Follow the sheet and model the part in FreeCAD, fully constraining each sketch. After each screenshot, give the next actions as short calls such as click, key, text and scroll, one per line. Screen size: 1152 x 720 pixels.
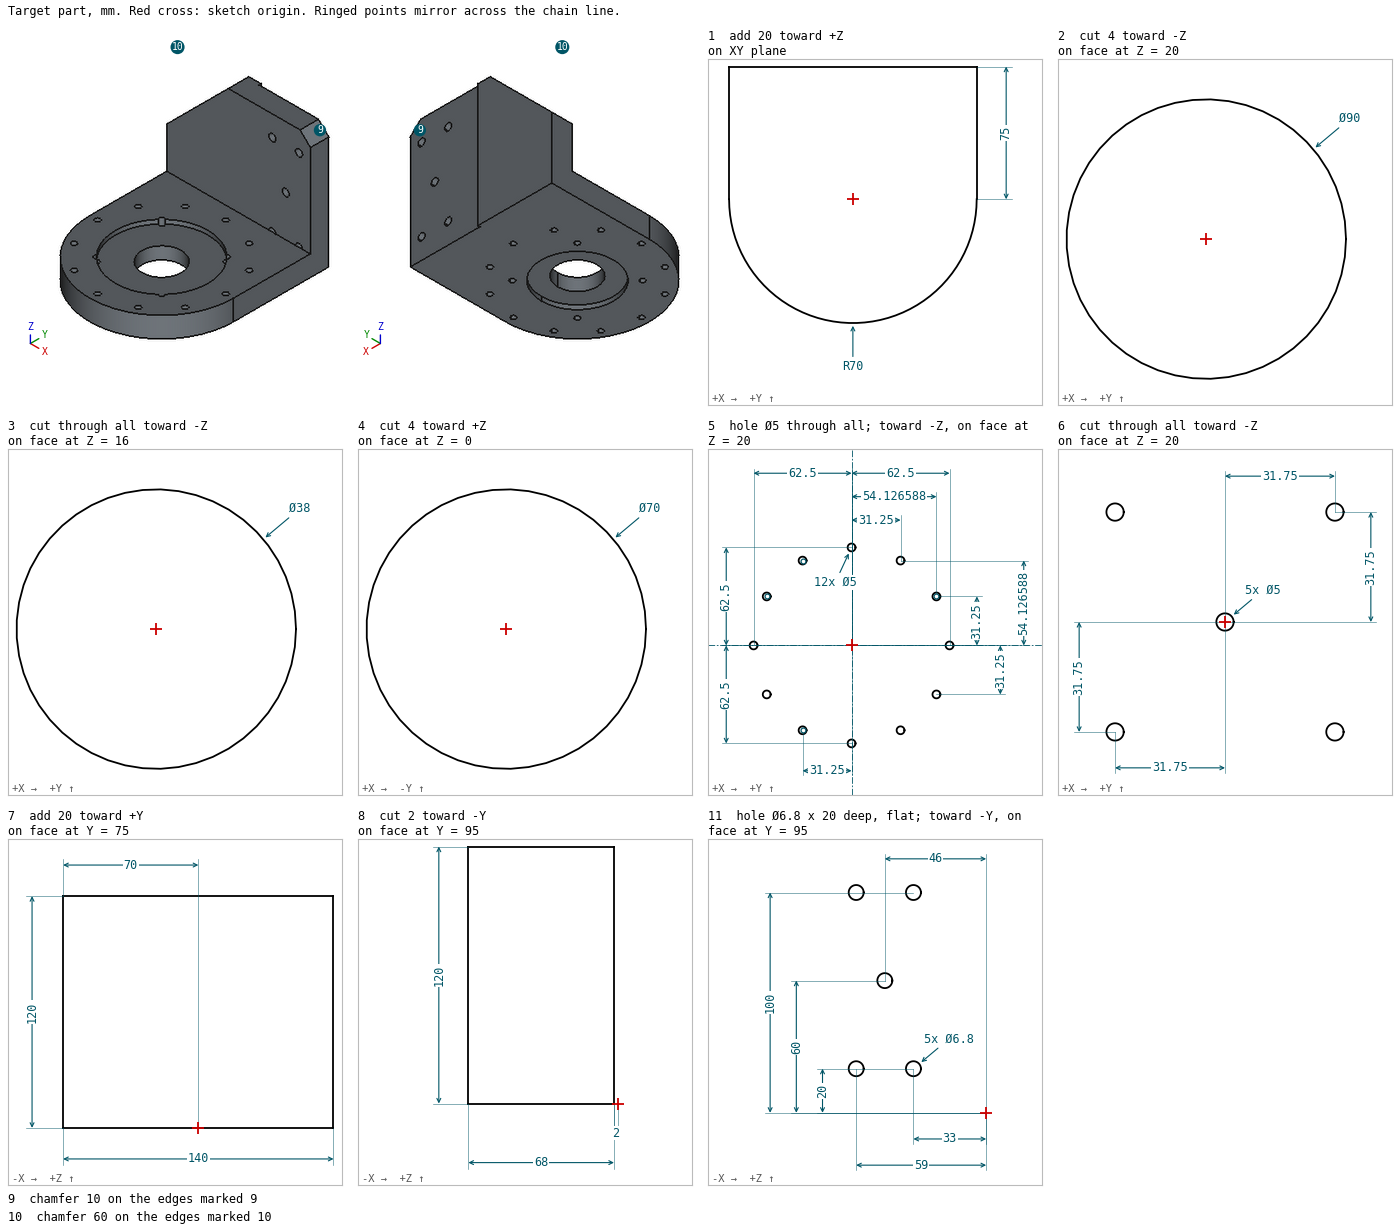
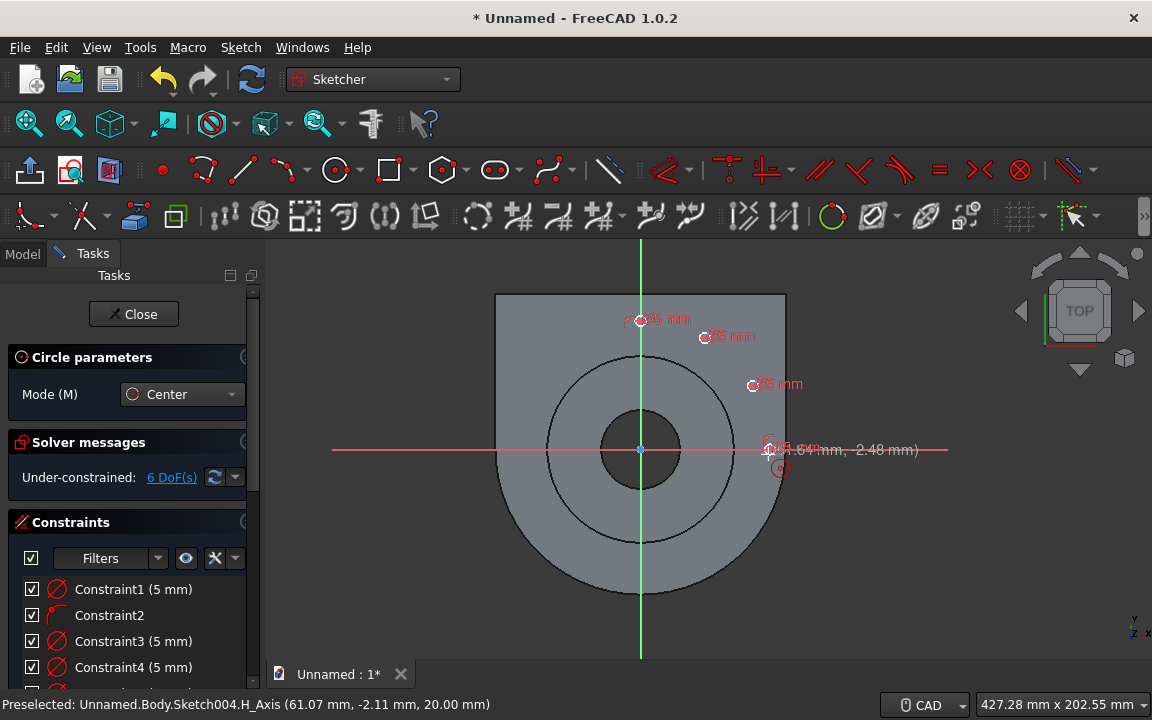
scroll(753, 514, up, 8)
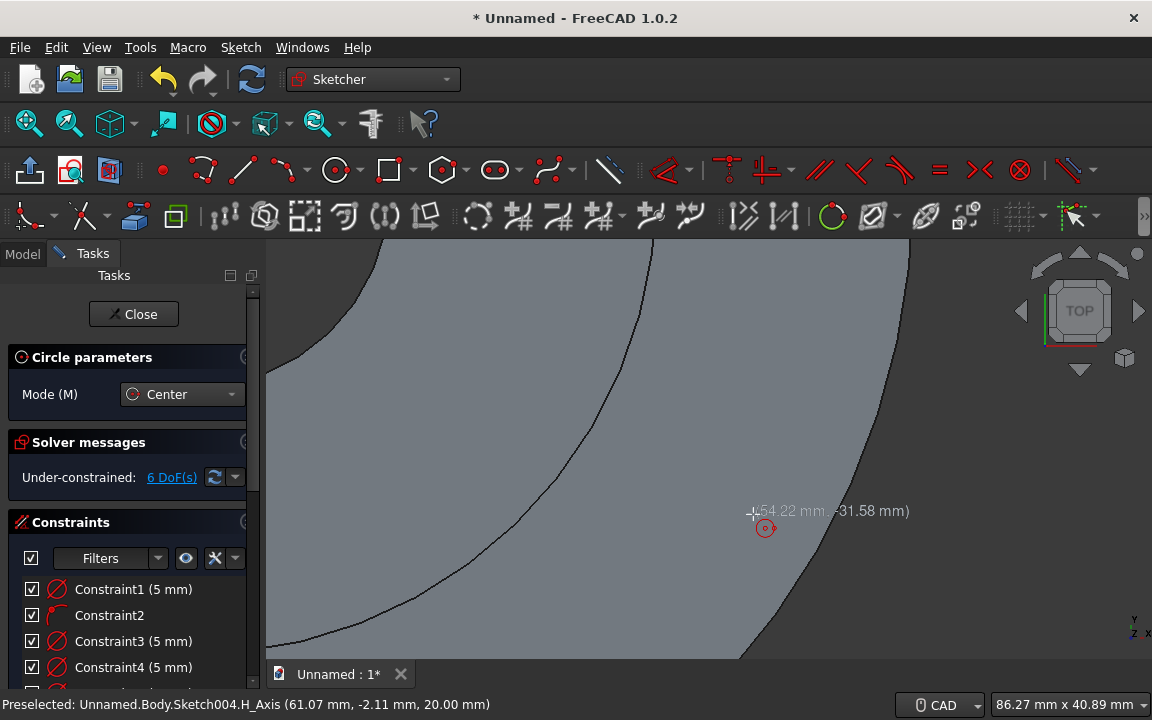
scroll(753, 514, down, 8)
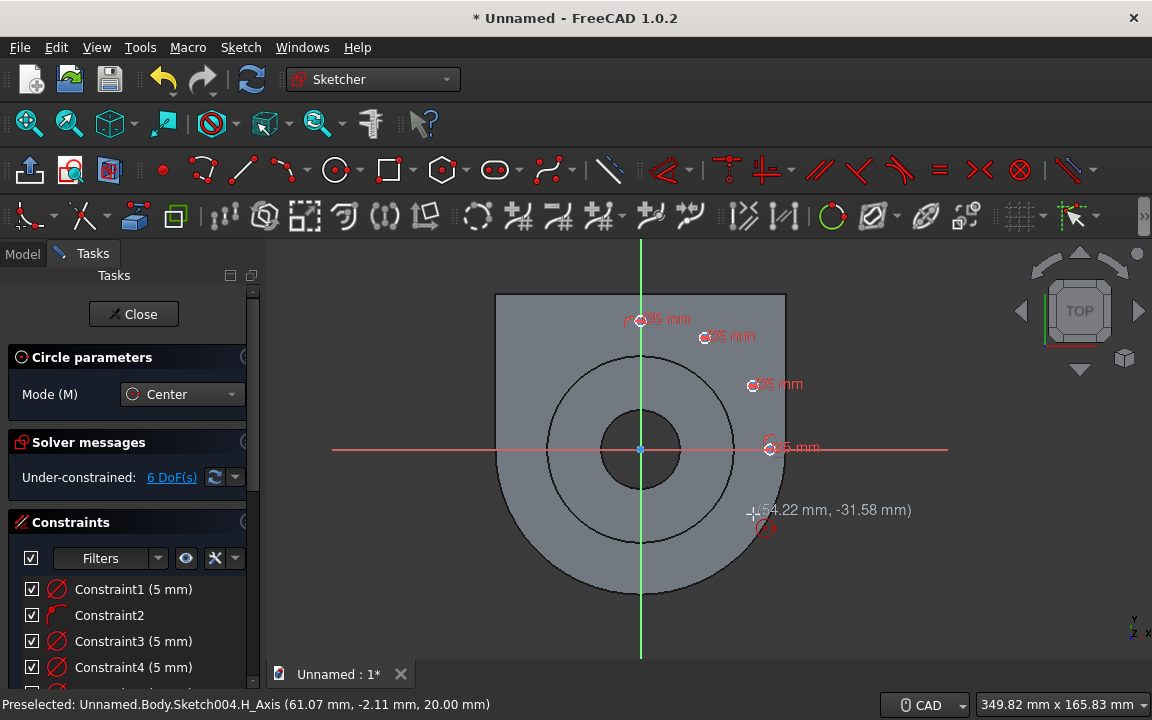
click(753, 514)
move(756, 511)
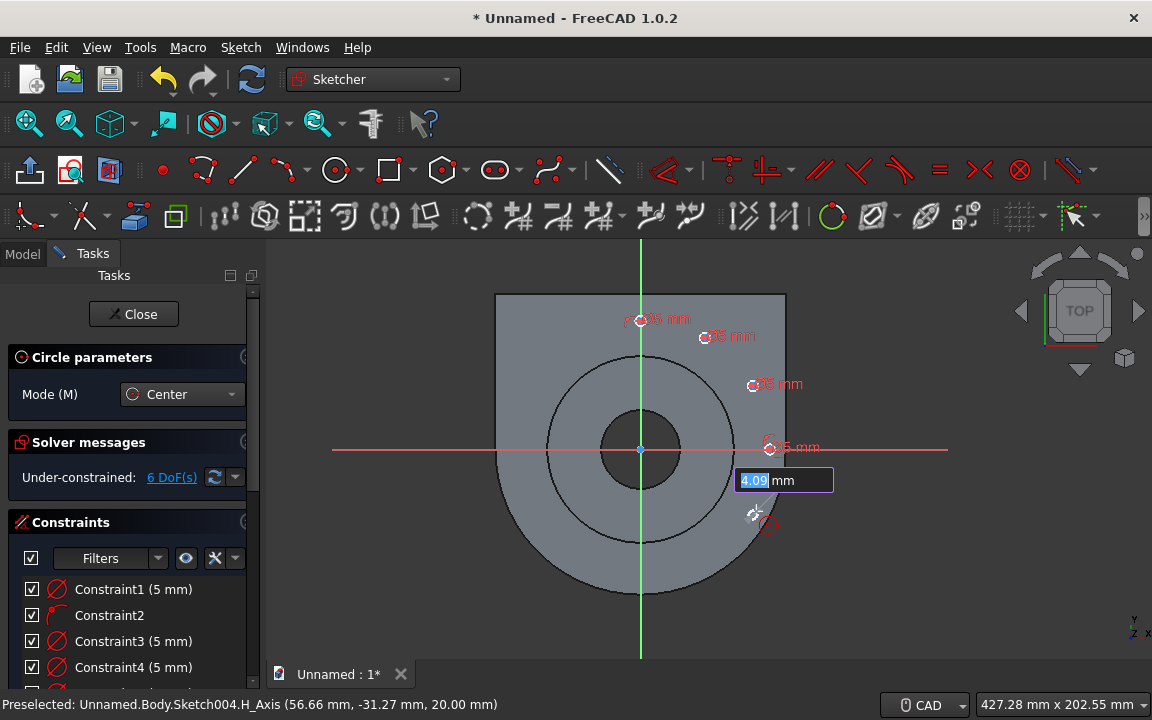
text(5)
key(Return)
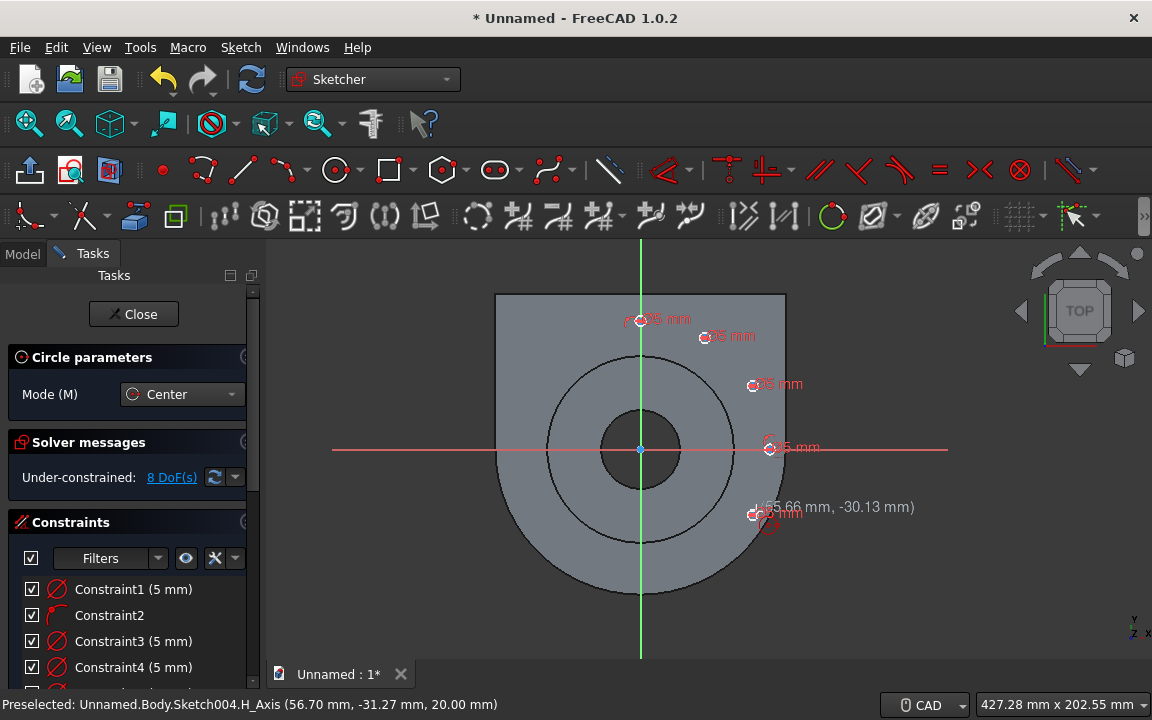
scroll(705, 562, up, 8)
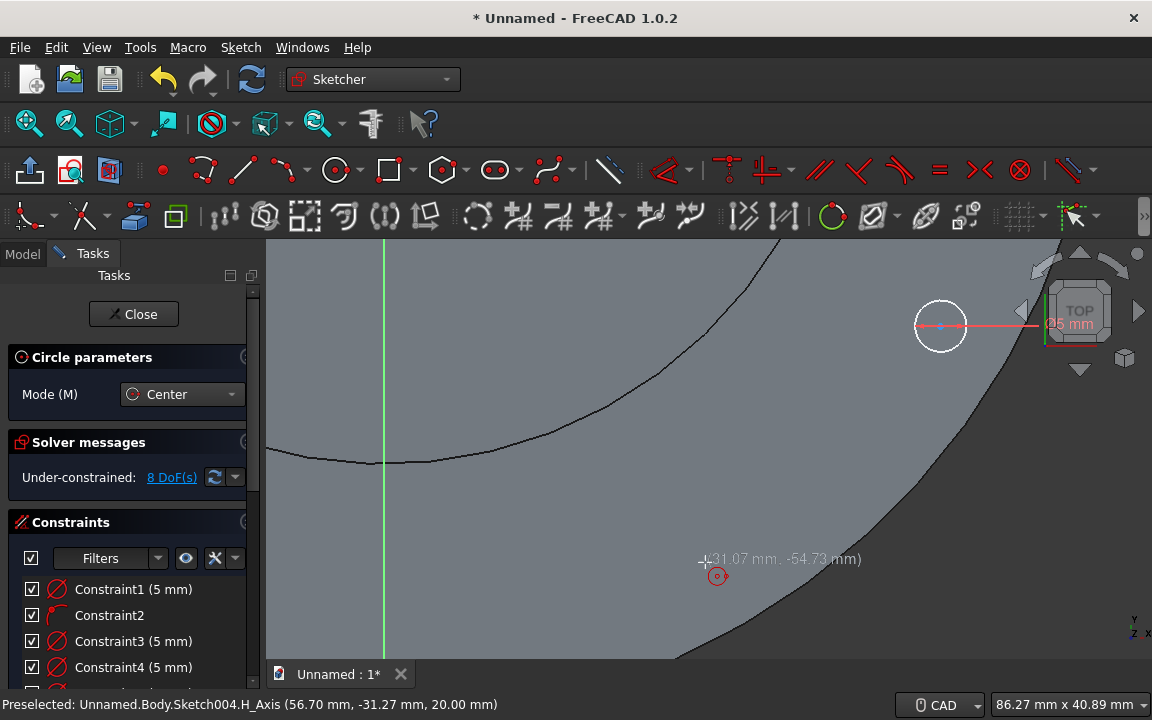
scroll(705, 562, down, 8)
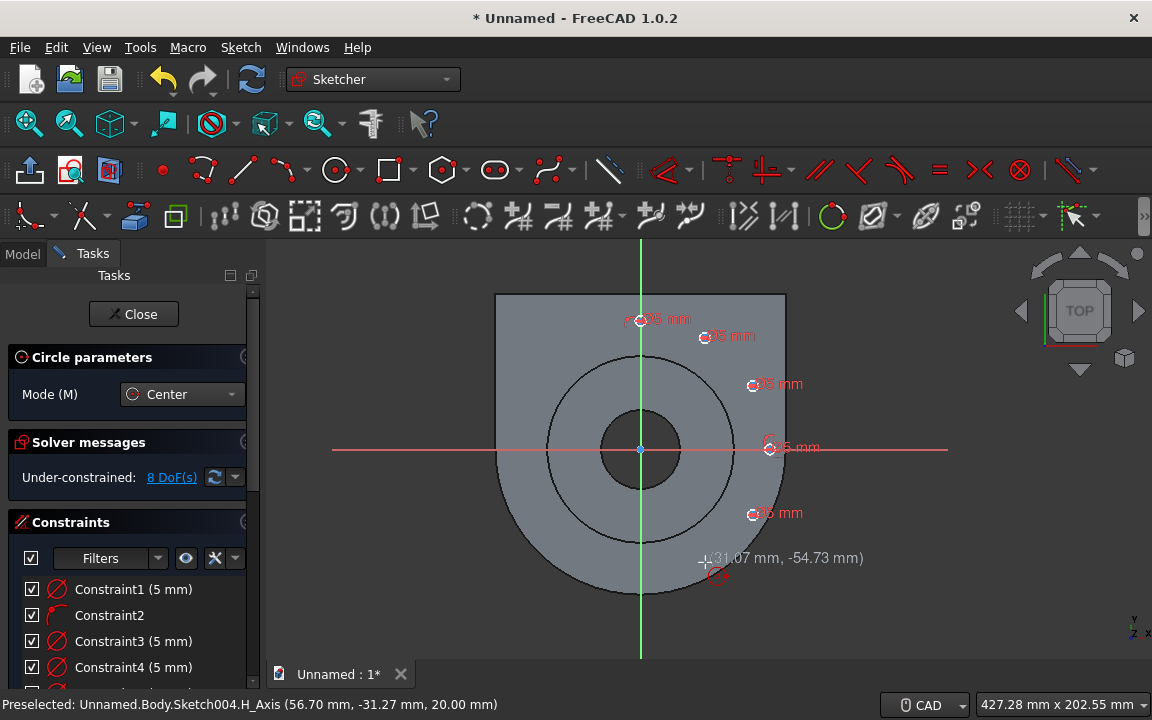
click(705, 562)
move(709, 558)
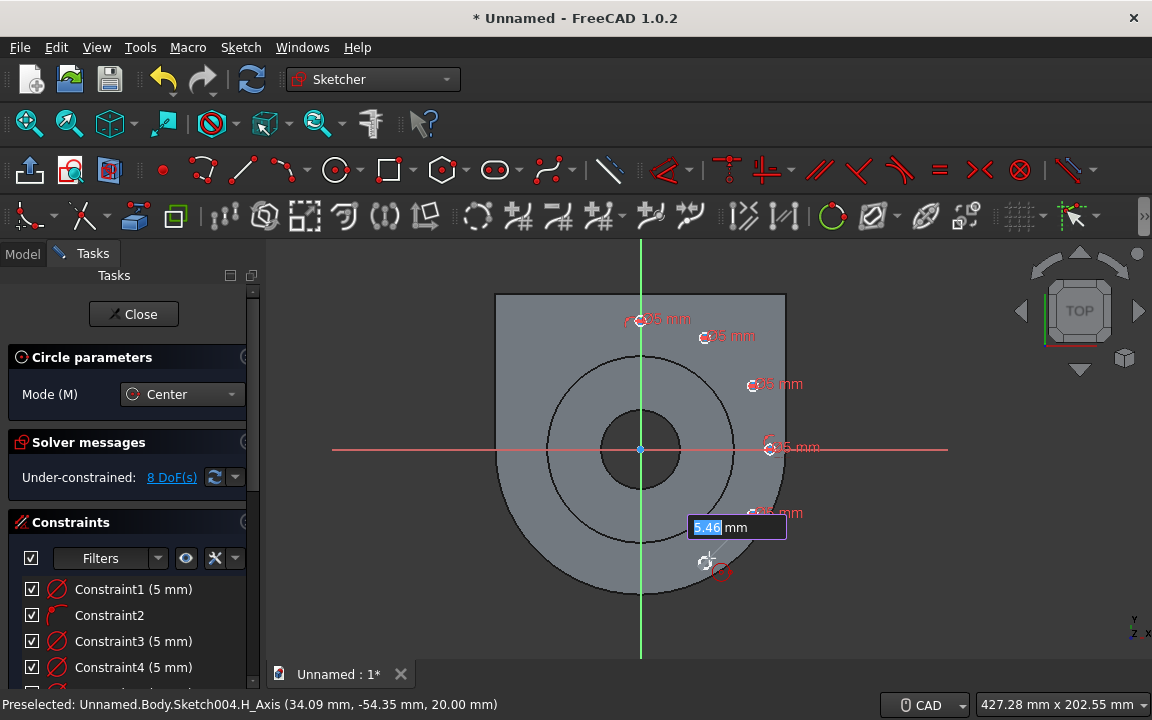
text(5)
key(Return)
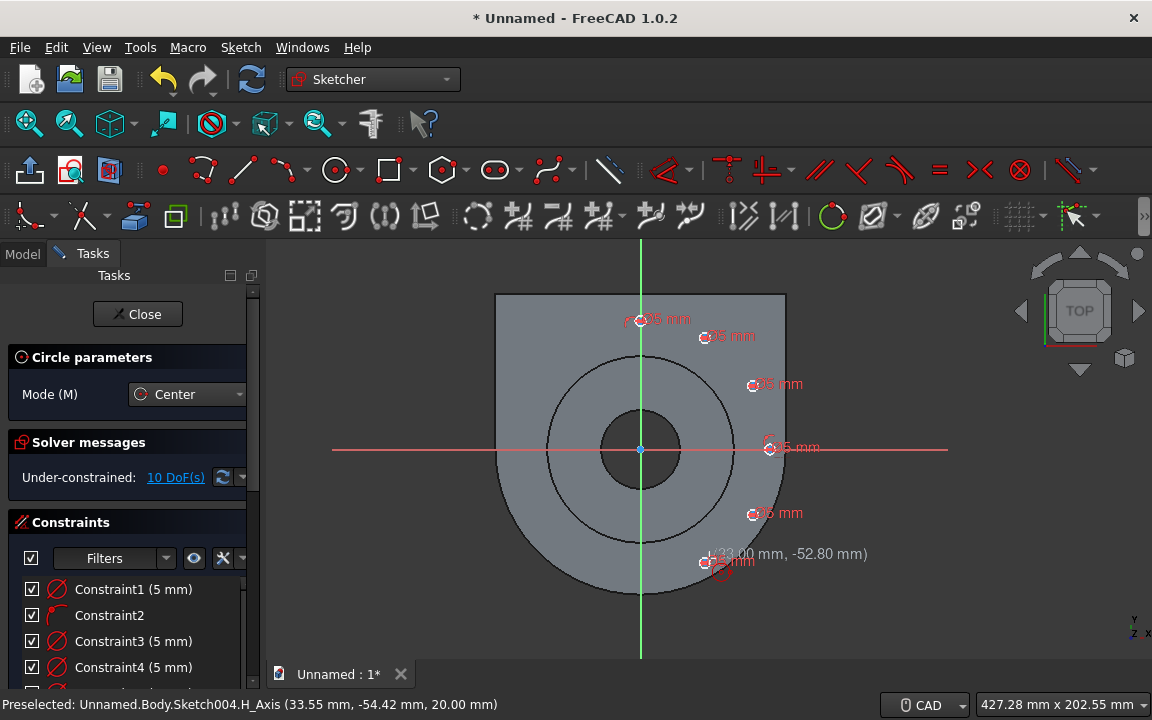
scroll(641, 579, up, 8)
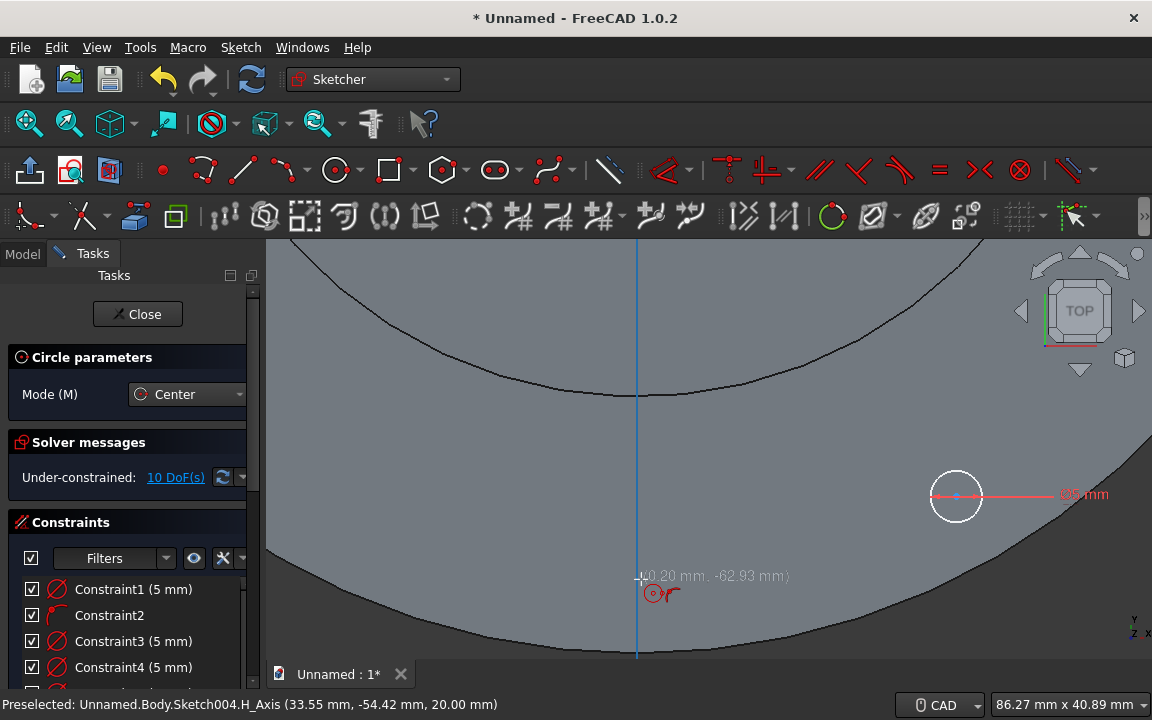
scroll(641, 579, down, 8)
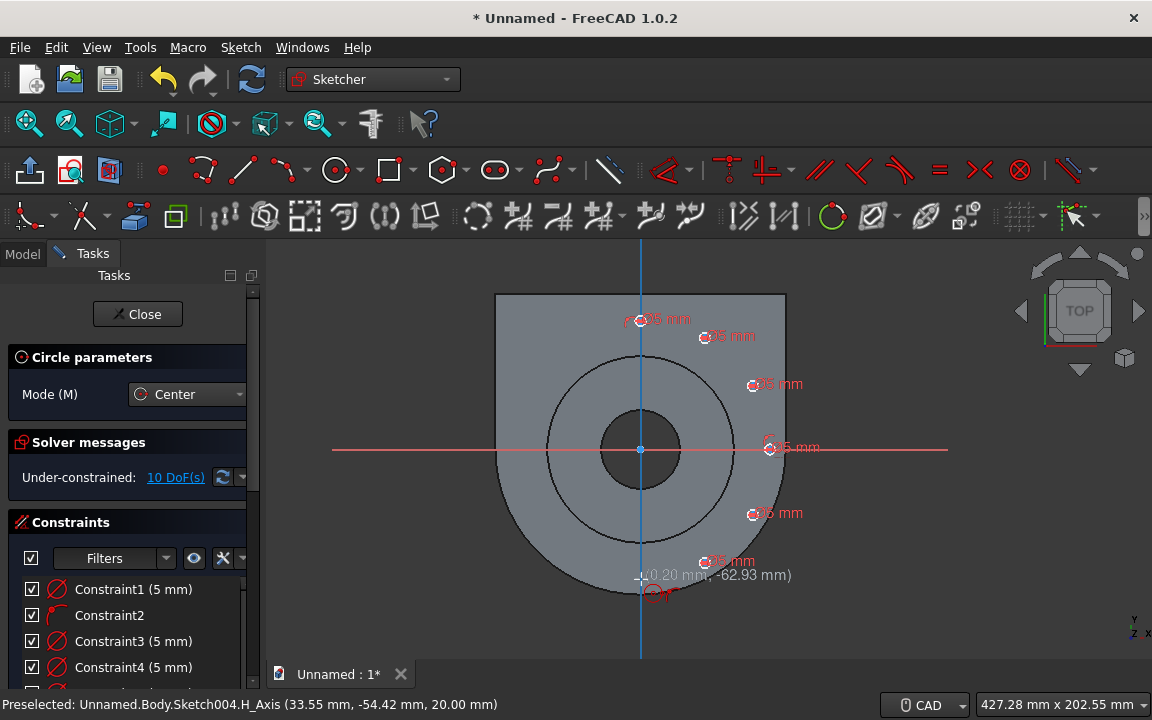
click(641, 579)